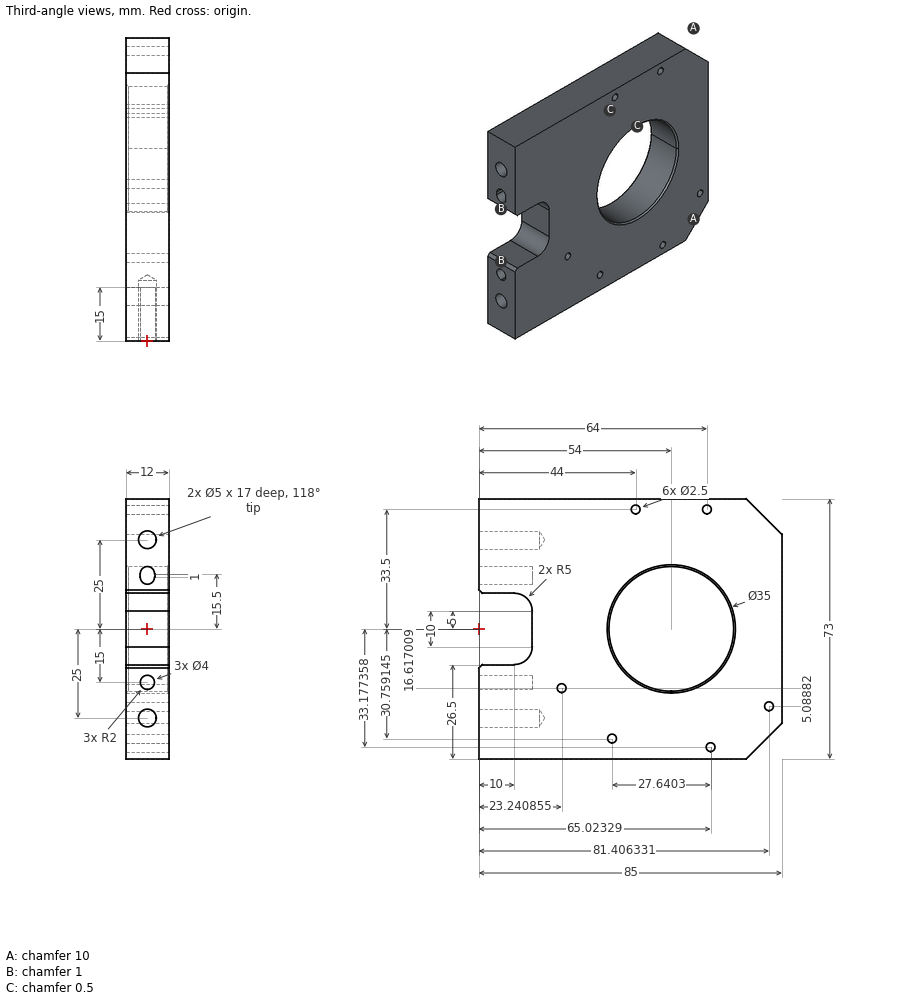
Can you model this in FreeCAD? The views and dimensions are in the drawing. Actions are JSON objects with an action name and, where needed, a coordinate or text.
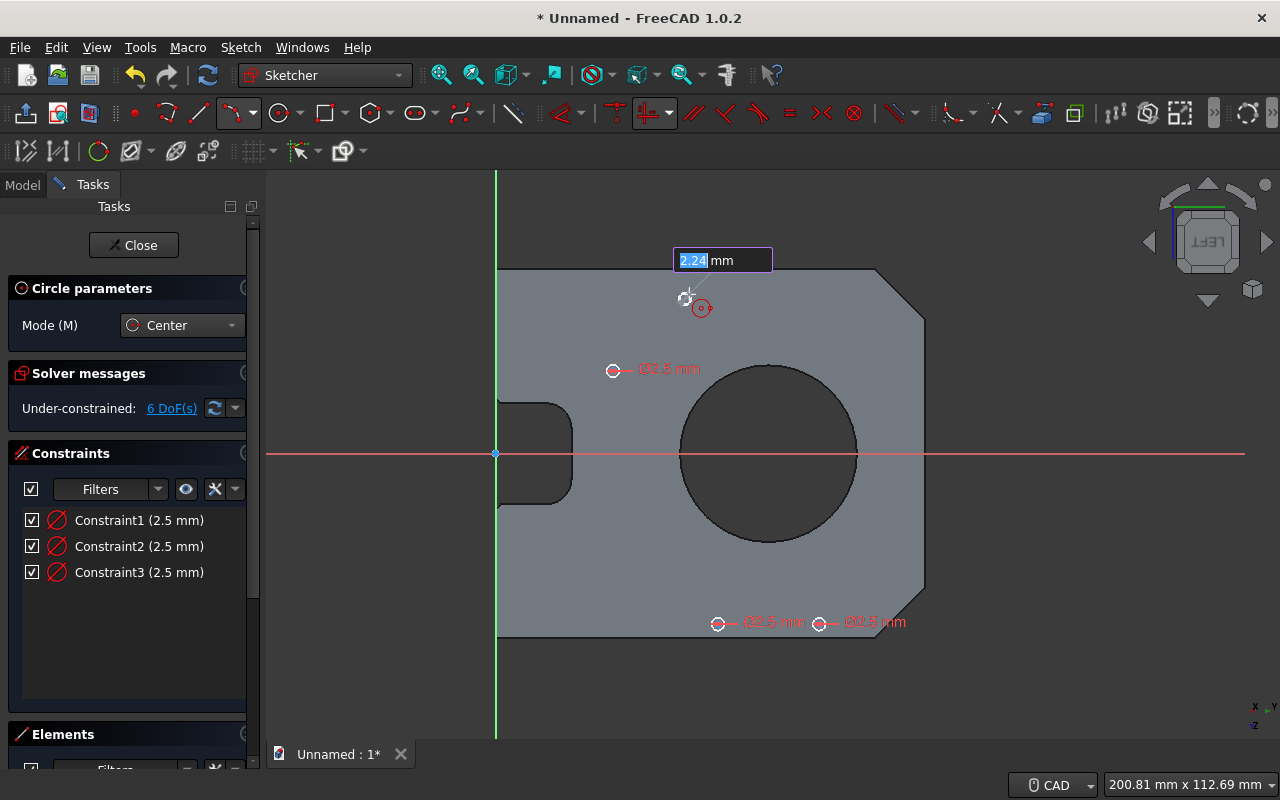
{"action": "type", "text": "2.5"}
{"action": "key", "text": "Return"}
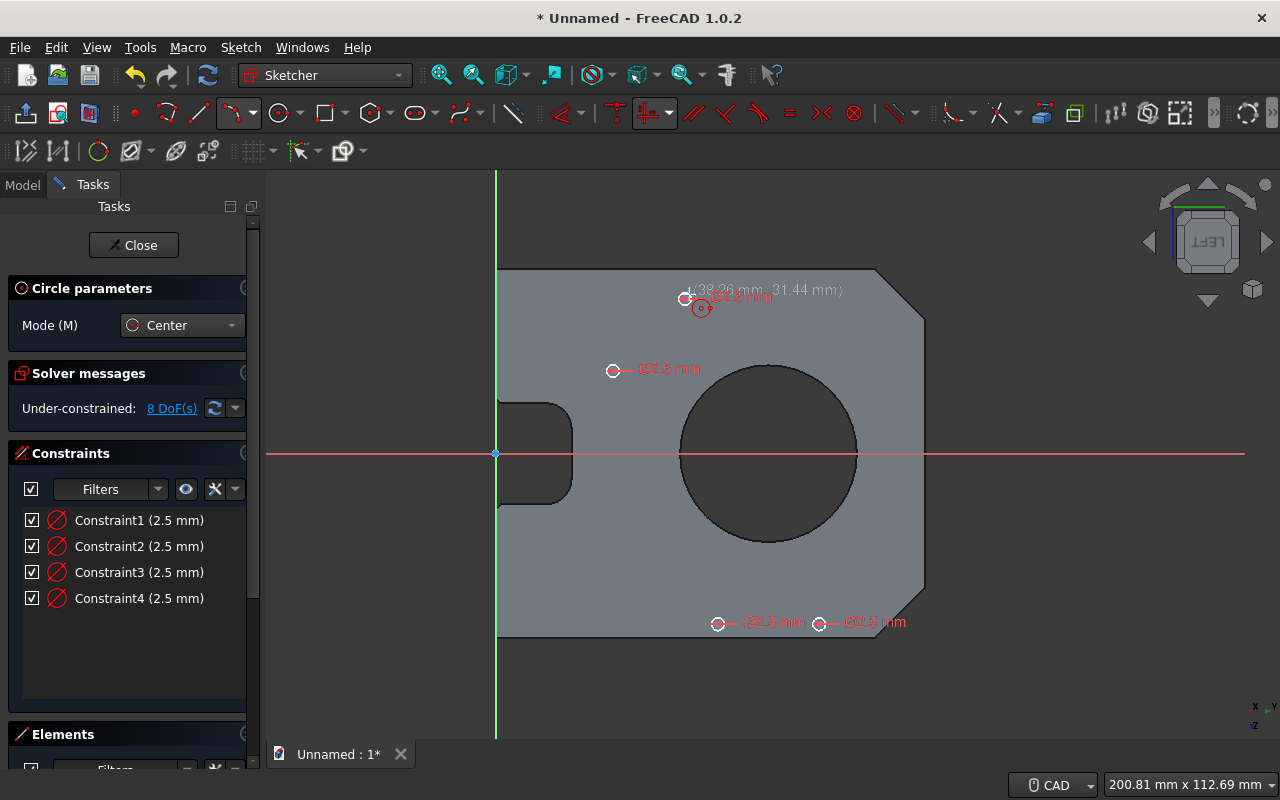
{"action": "scroll", "coordinate": [824, 286], "scroll_direction": "up", "scroll_amount": 7}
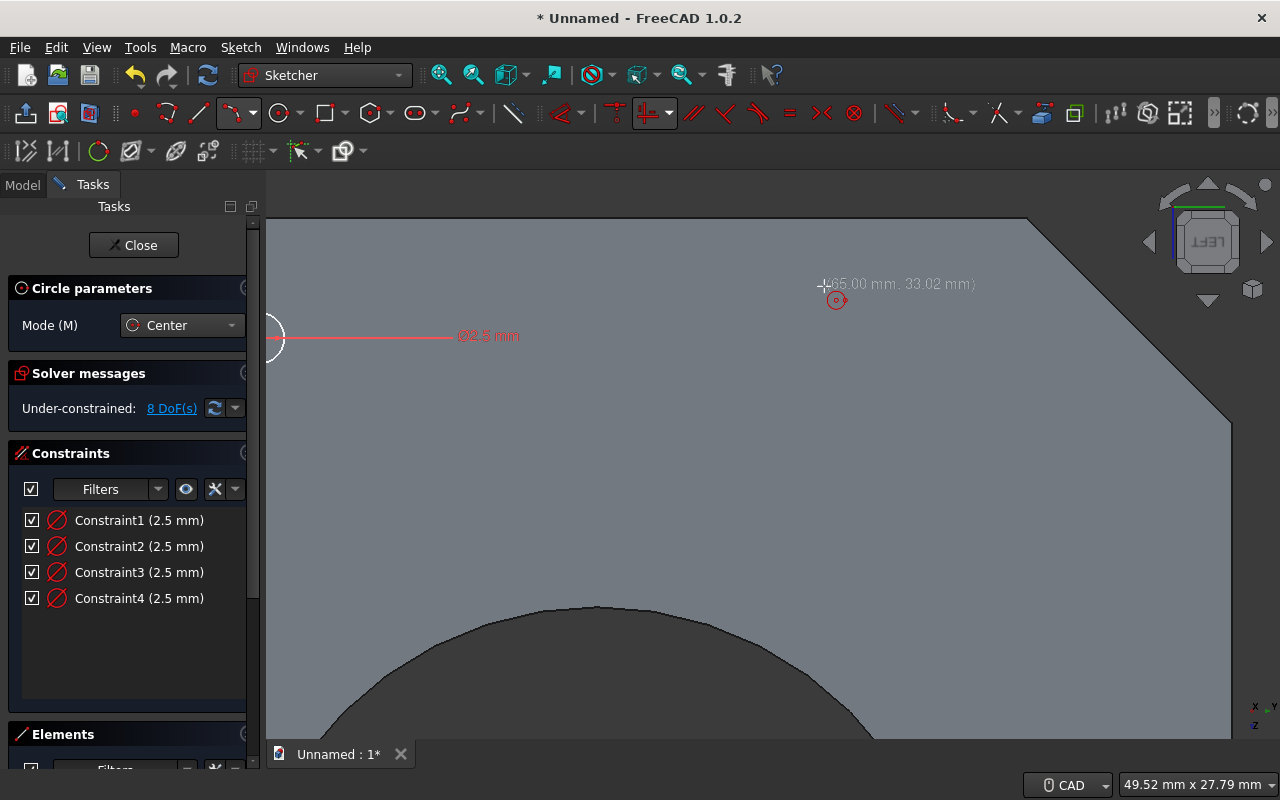
{"action": "scroll", "coordinate": [825, 286], "scroll_direction": "down", "scroll_amount": 7}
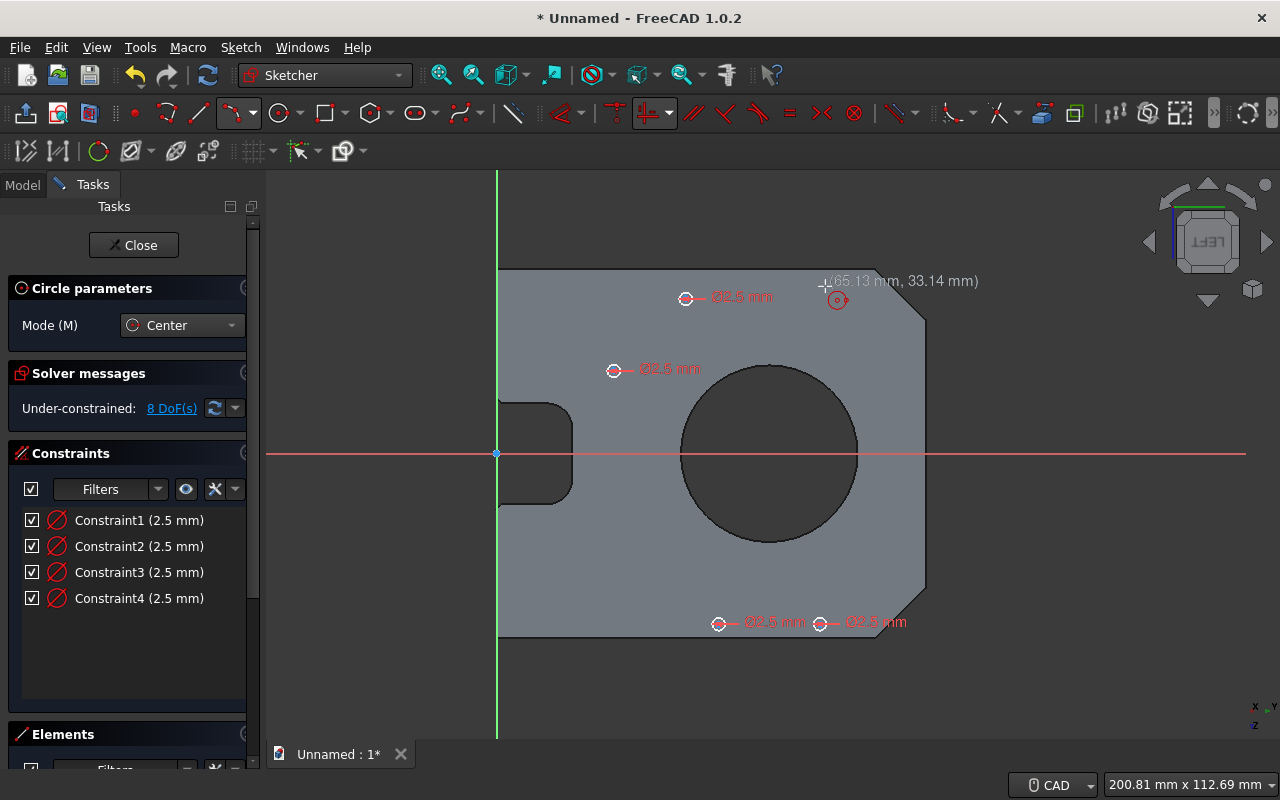
{"action": "left_click", "coordinate": [825, 286]}
{"action": "mouse_move", "coordinate": [829, 282]}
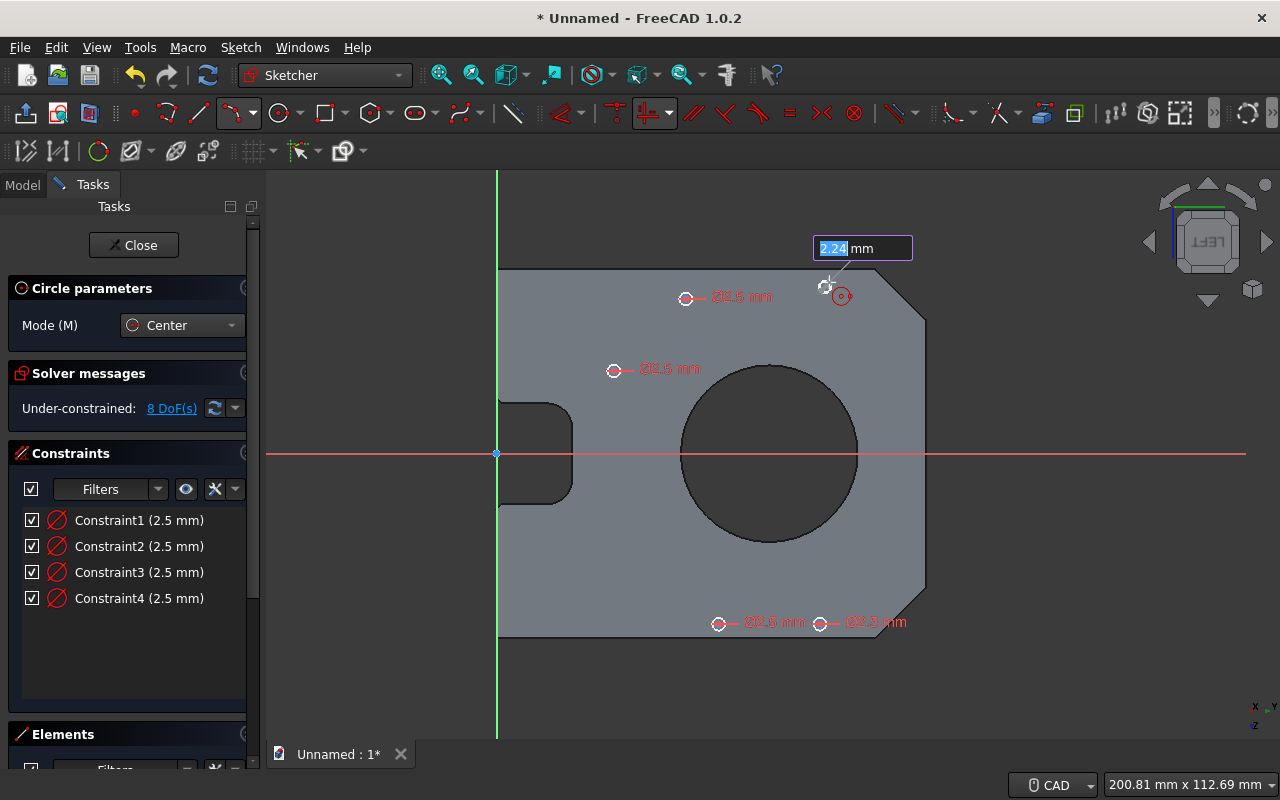
{"action": "type", "text": "2.5"}
{"action": "key", "text": "Return"}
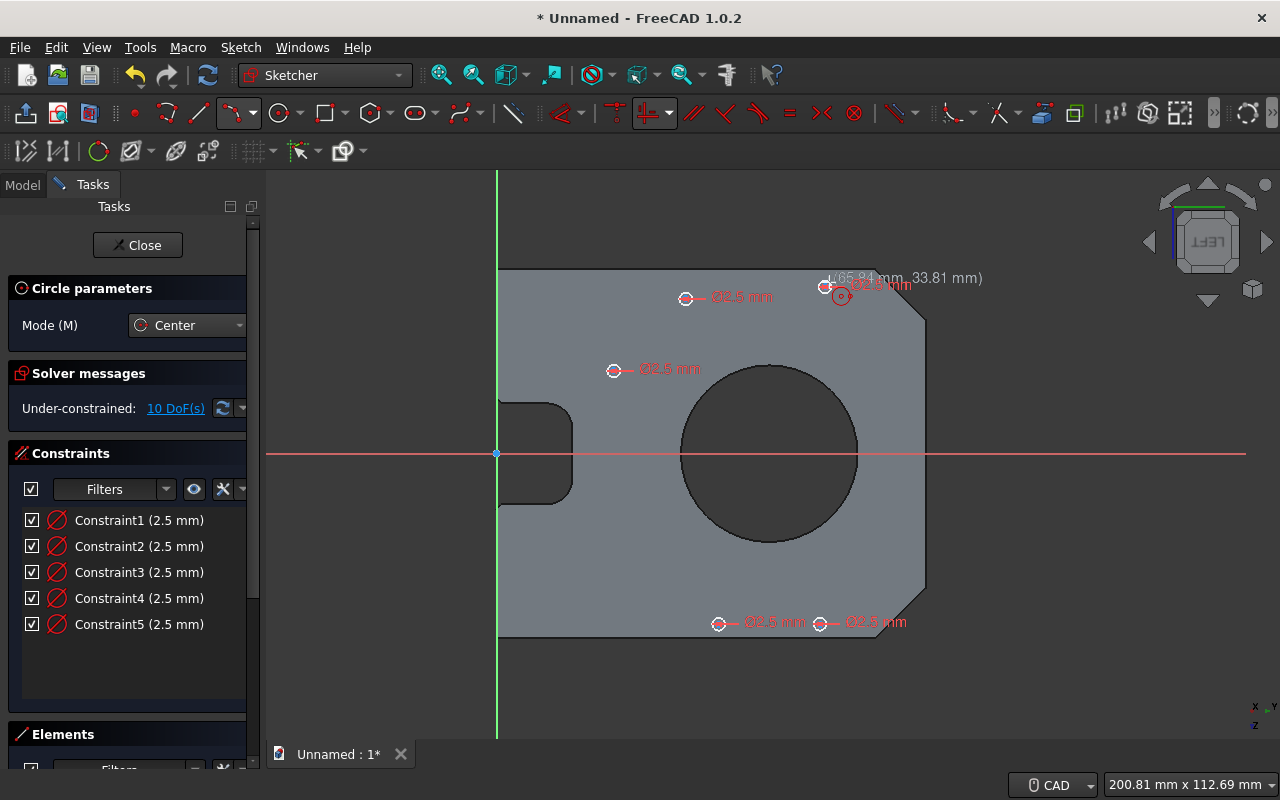
{"action": "scroll", "coordinate": [908, 344], "scroll_direction": "up", "scroll_amount": 7}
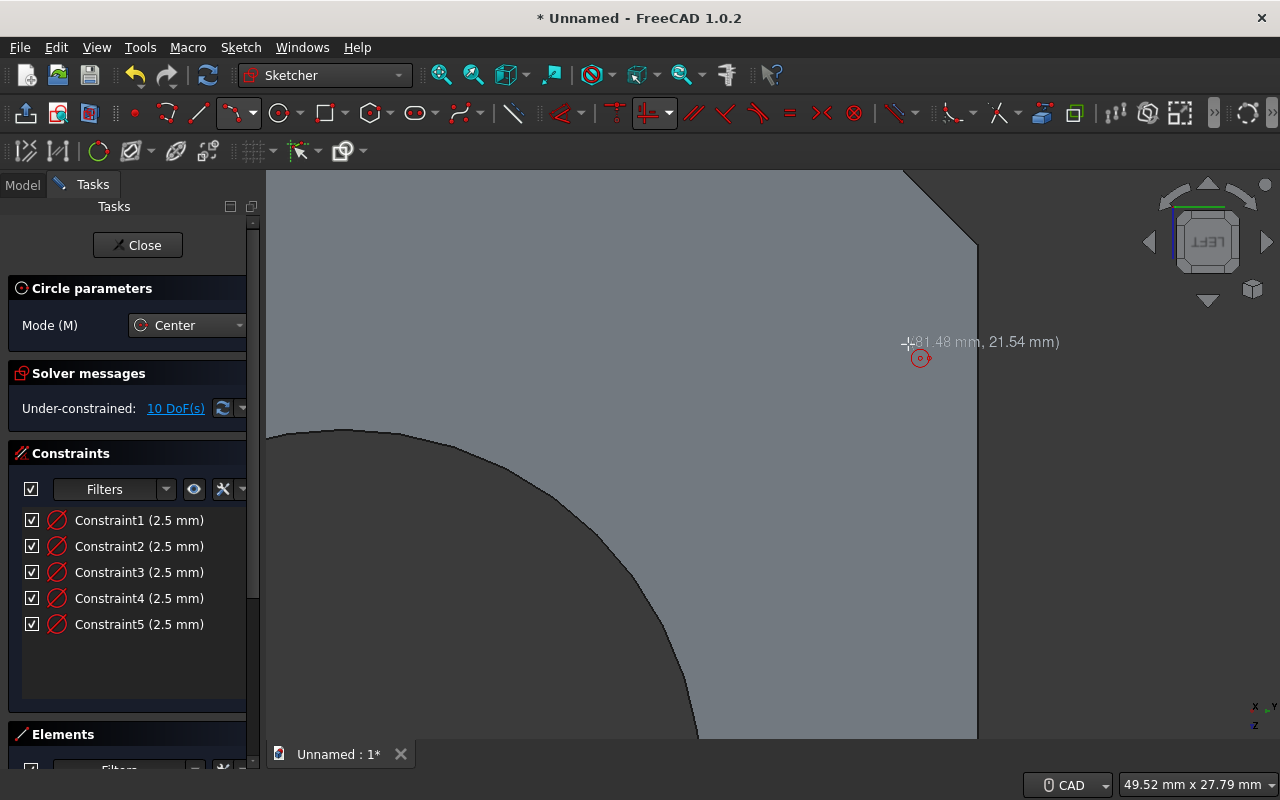
{"action": "scroll", "coordinate": [908, 344], "scroll_direction": "down", "scroll_amount": 7}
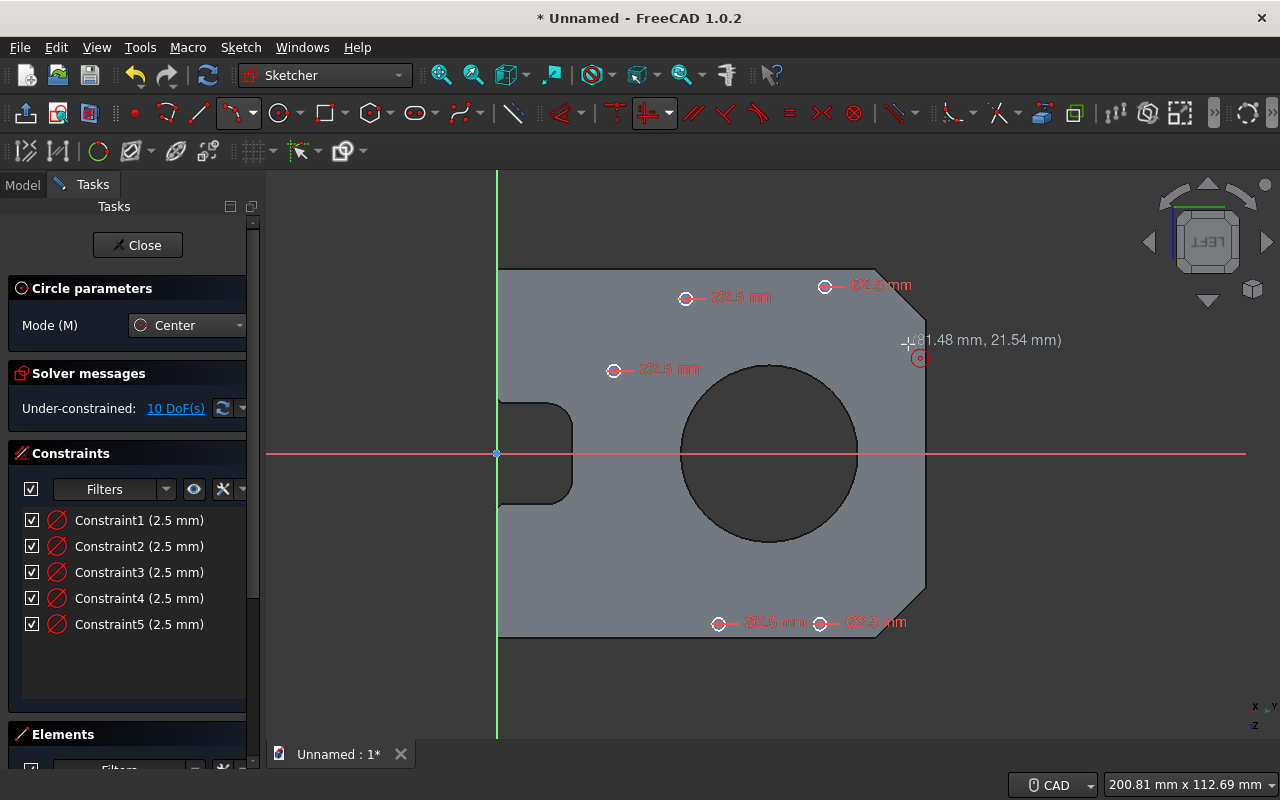
{"action": "left_click", "coordinate": [908, 344]}
{"action": "mouse_move", "coordinate": [912, 340]}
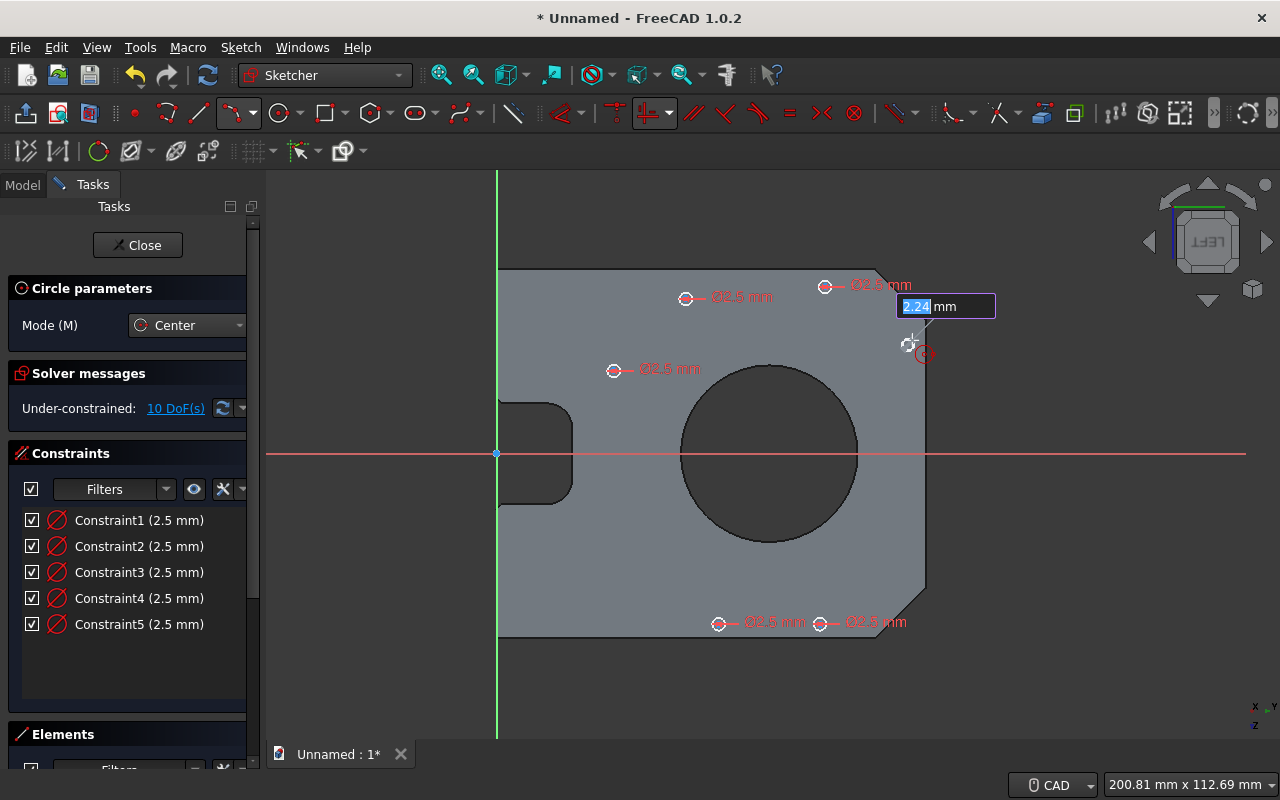
{"action": "type", "text": "2.5"}
{"action": "key", "text": "Return"}
{"action": "key", "text": "Escape"}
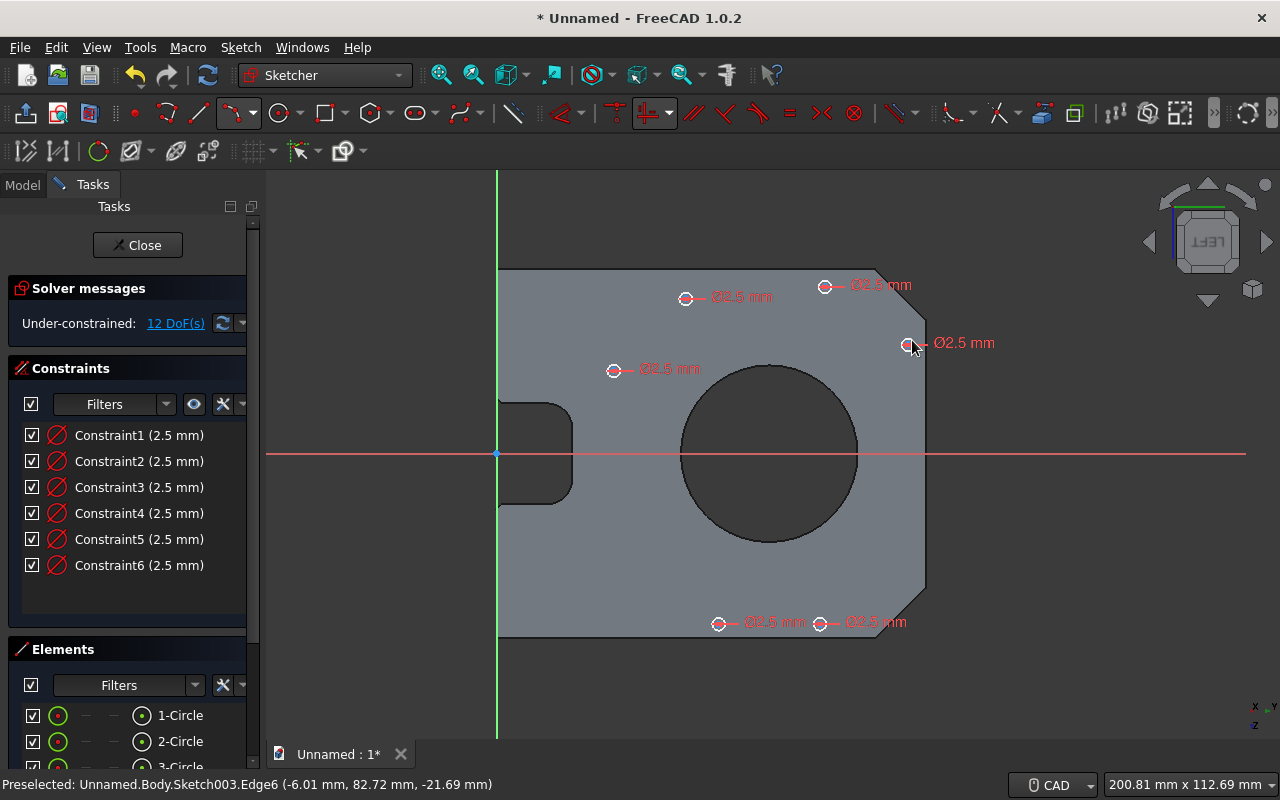
{"action": "left_click", "coordinate": [719, 624]}